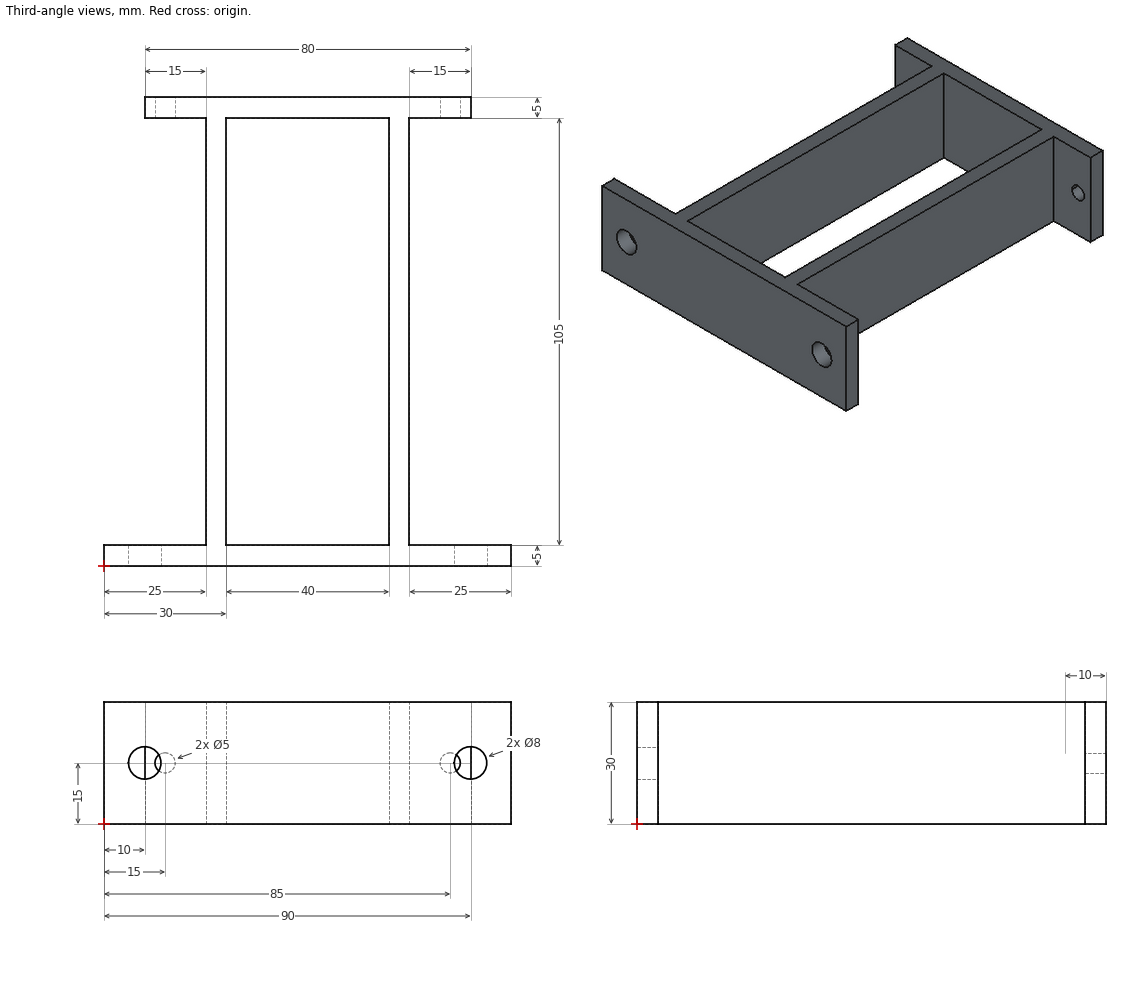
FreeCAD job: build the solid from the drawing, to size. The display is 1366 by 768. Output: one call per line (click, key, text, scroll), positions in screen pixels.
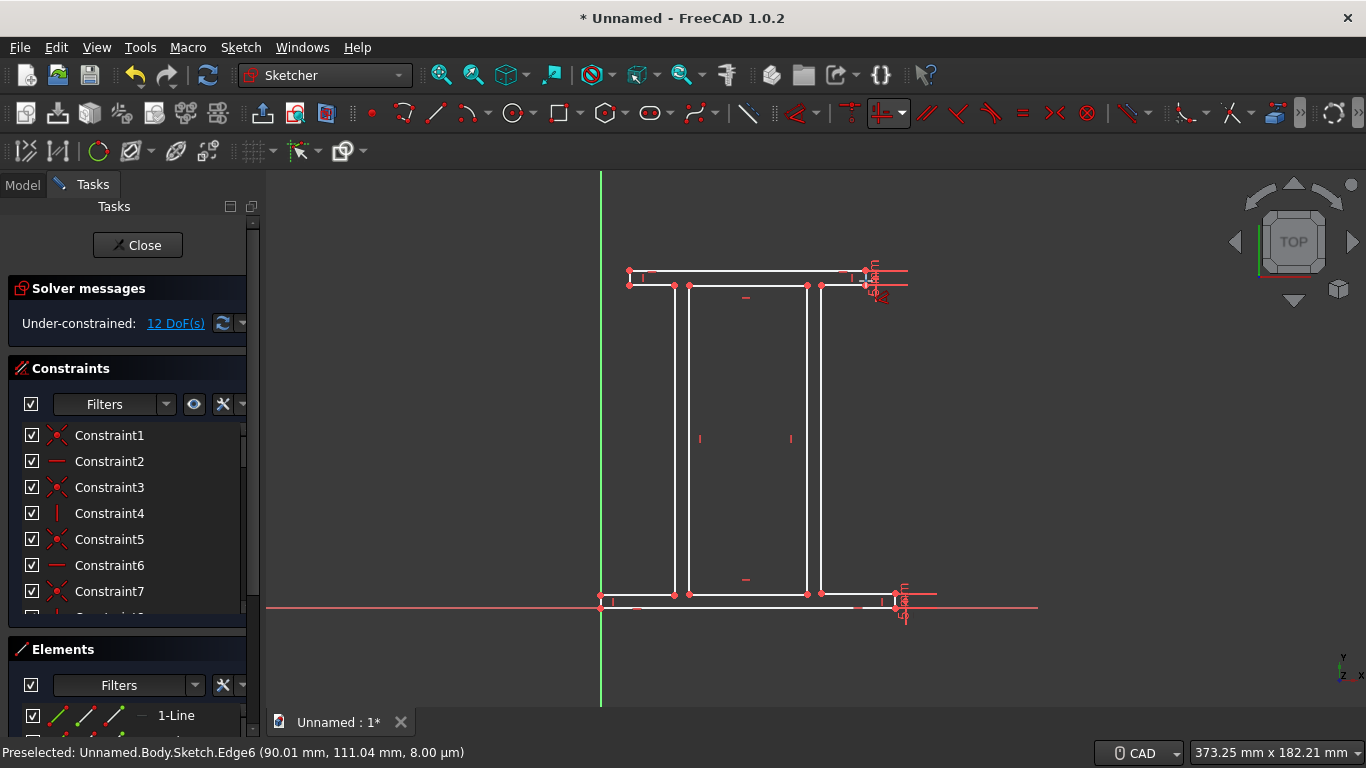
scroll(630, 275, up, 6)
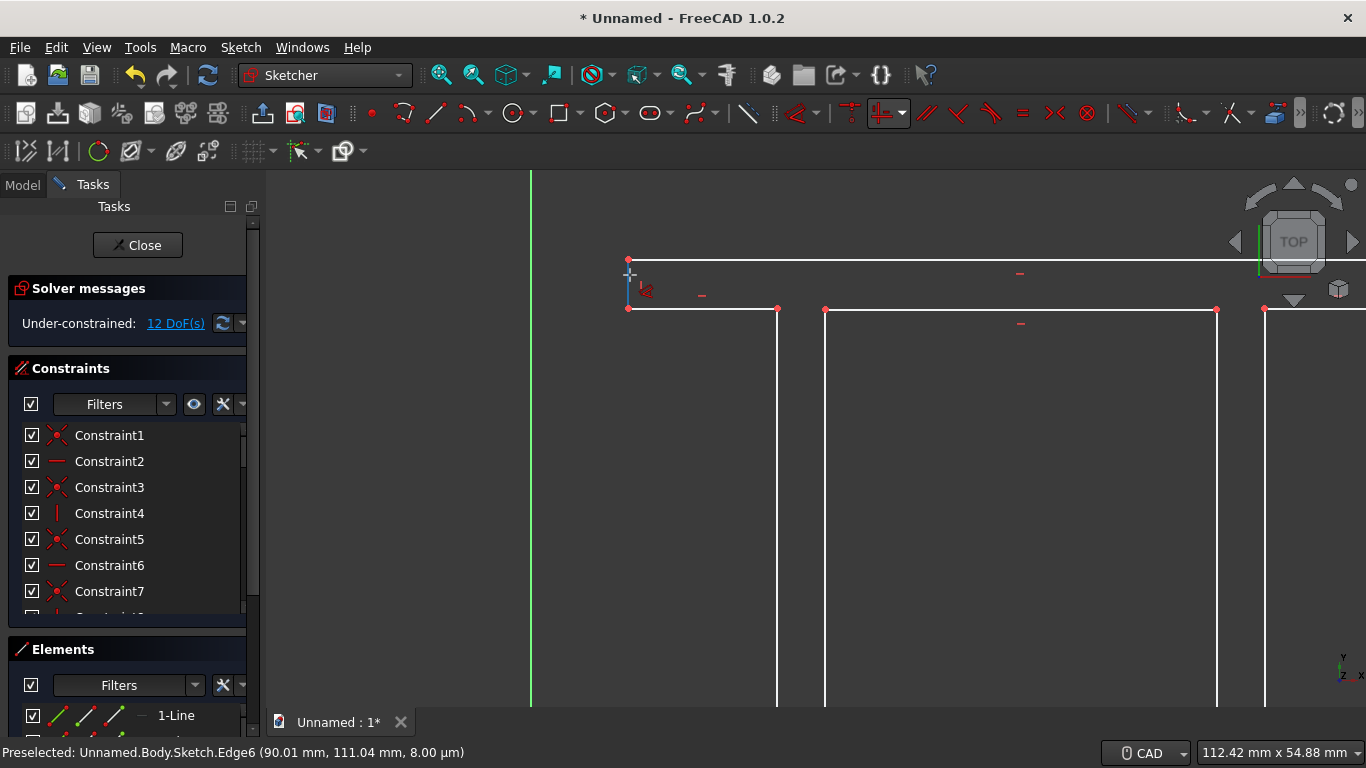
click(628, 274)
click(594, 284)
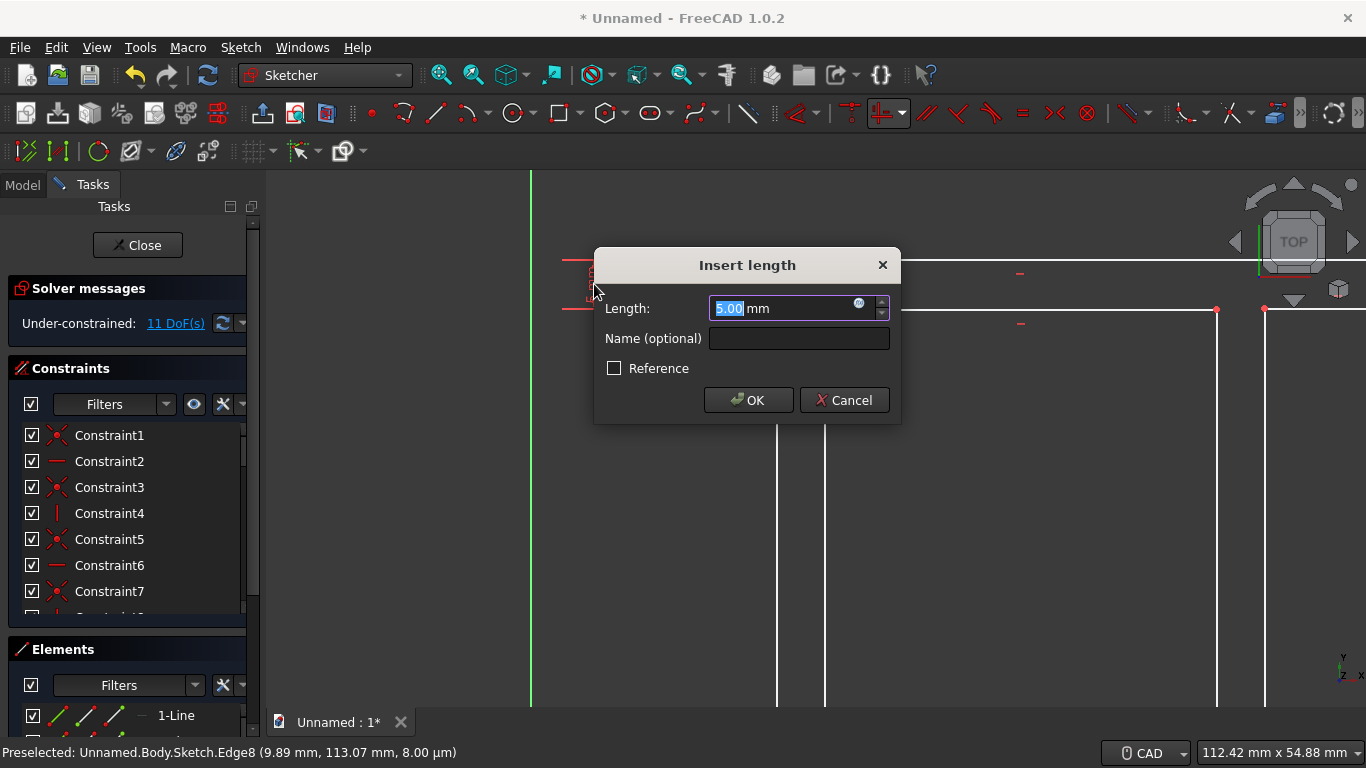
text(5)
key(Return)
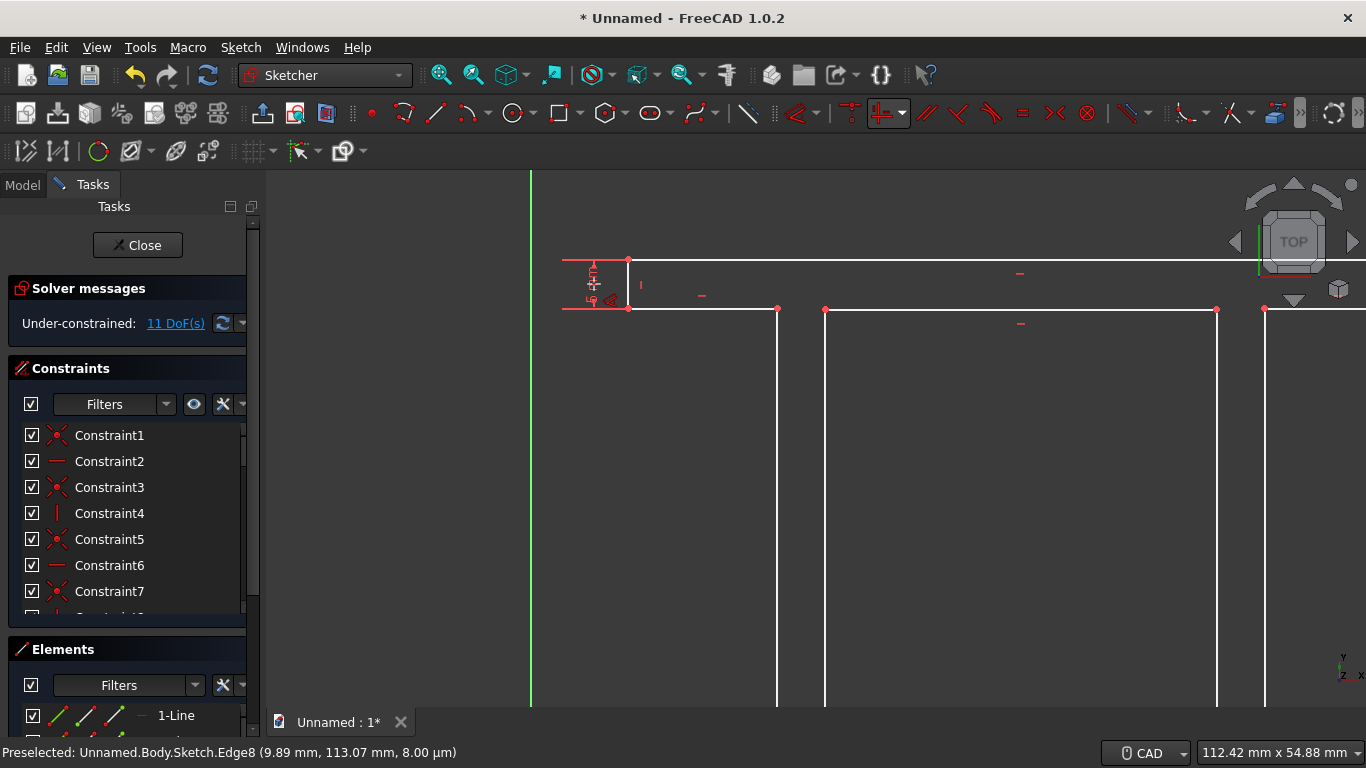
scroll(630, 275, down, 6)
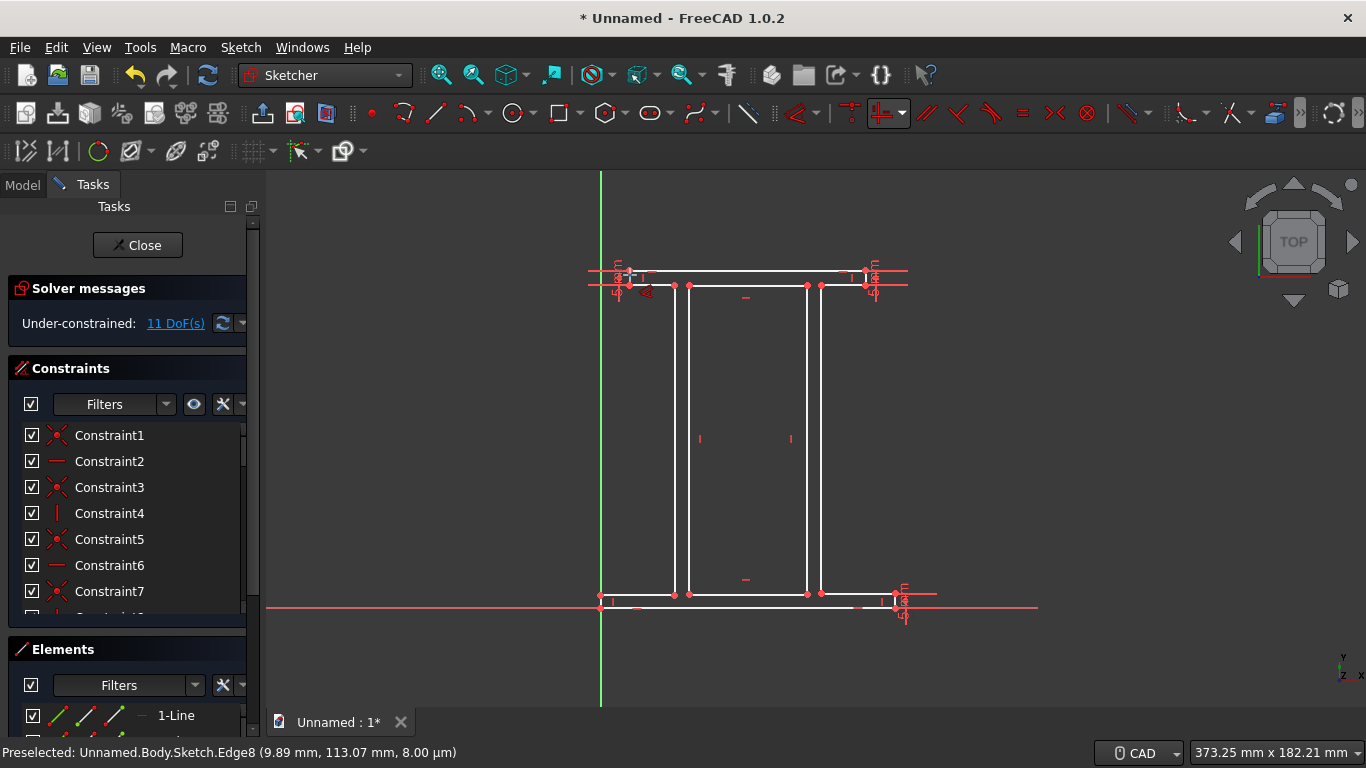
scroll(601, 599, up, 7)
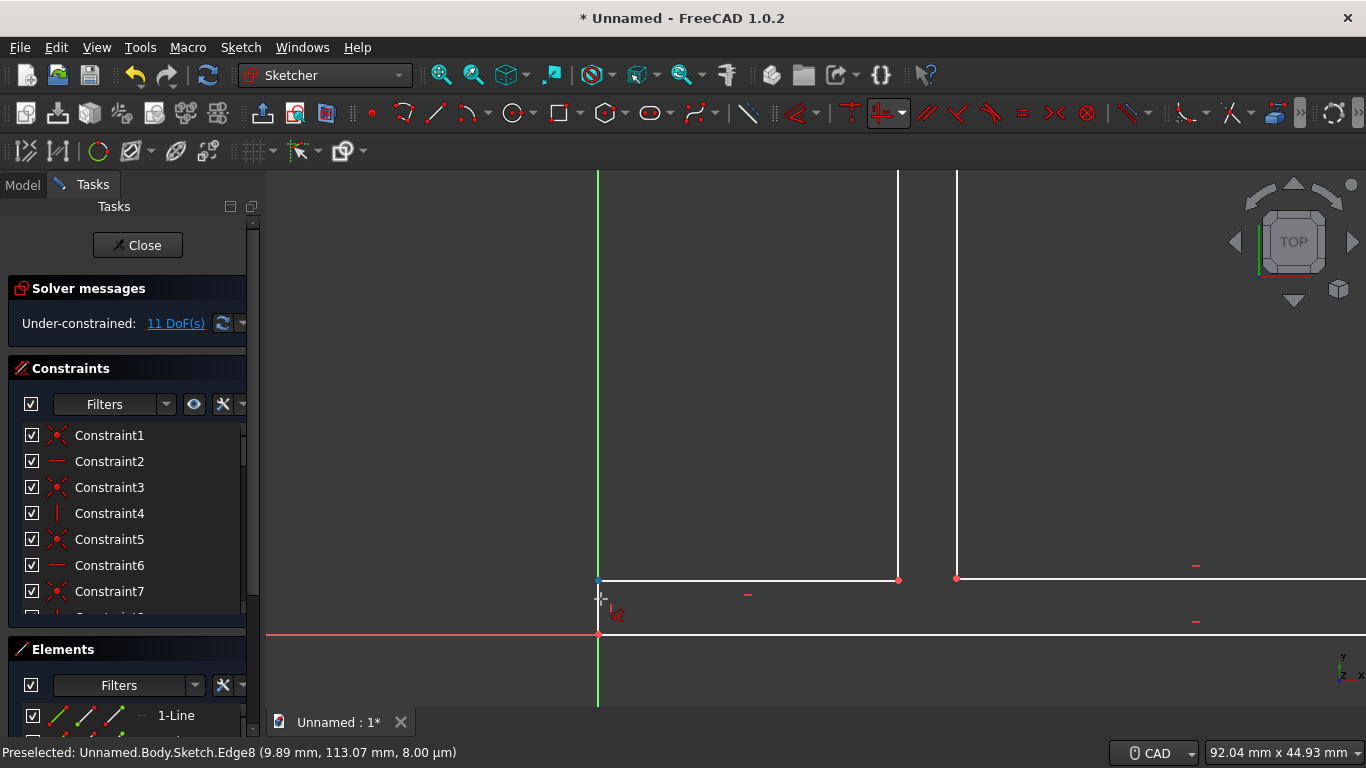
click(598, 597)
click(564, 608)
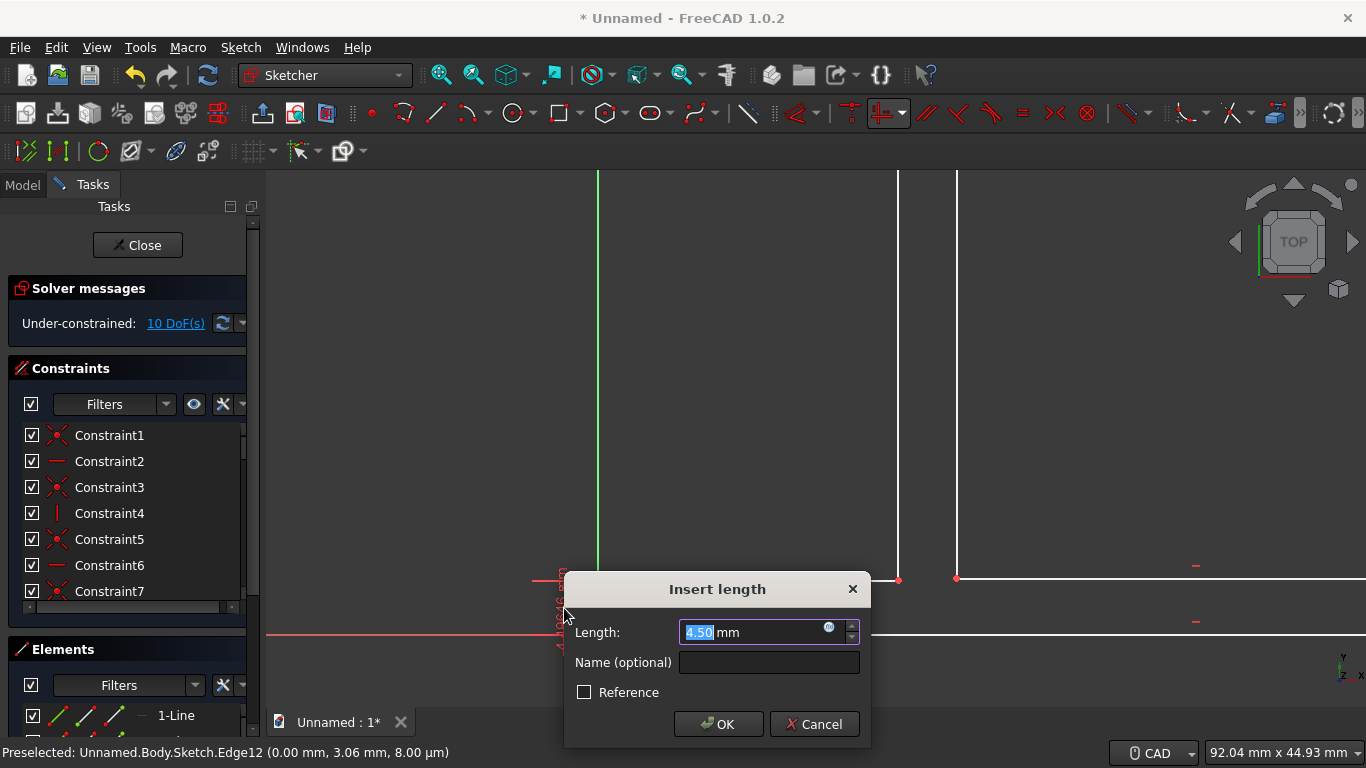
text(5)
key(Return)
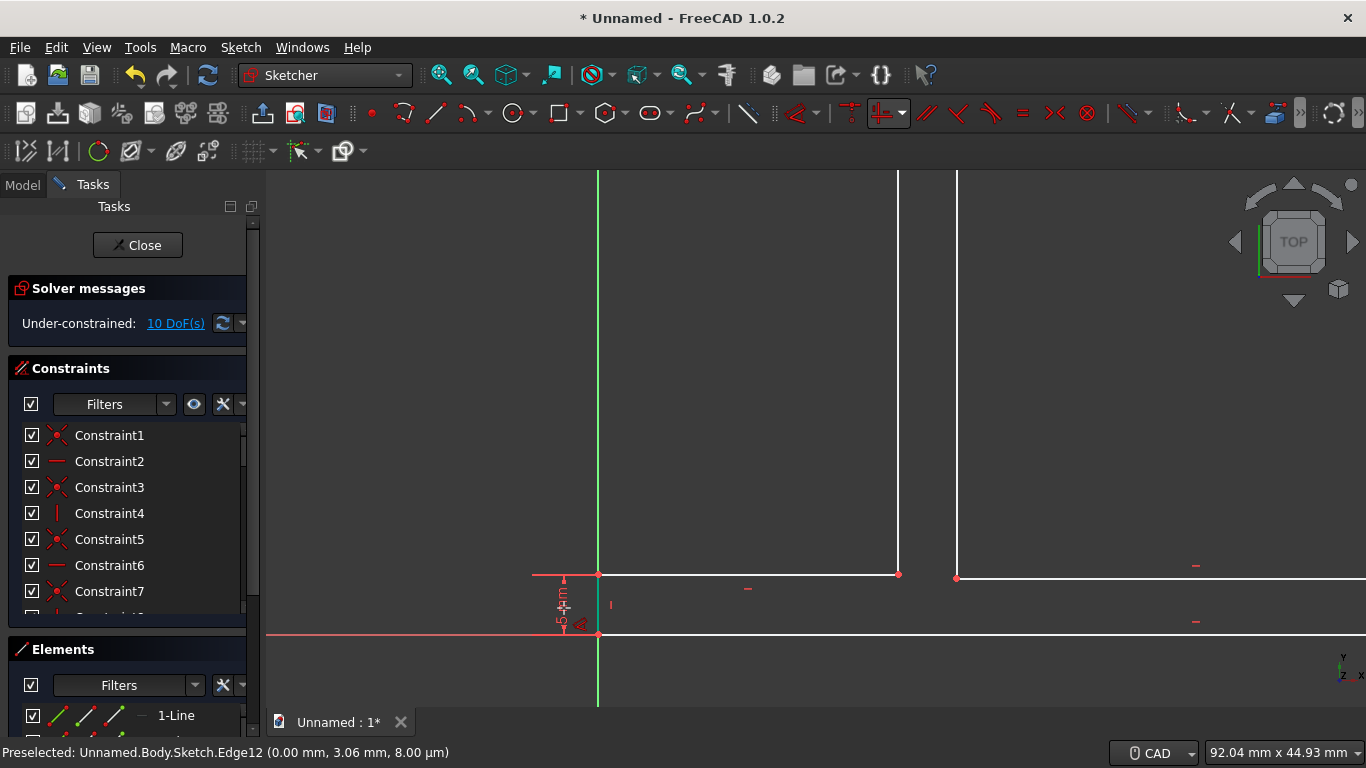
scroll(601, 599, down, 7)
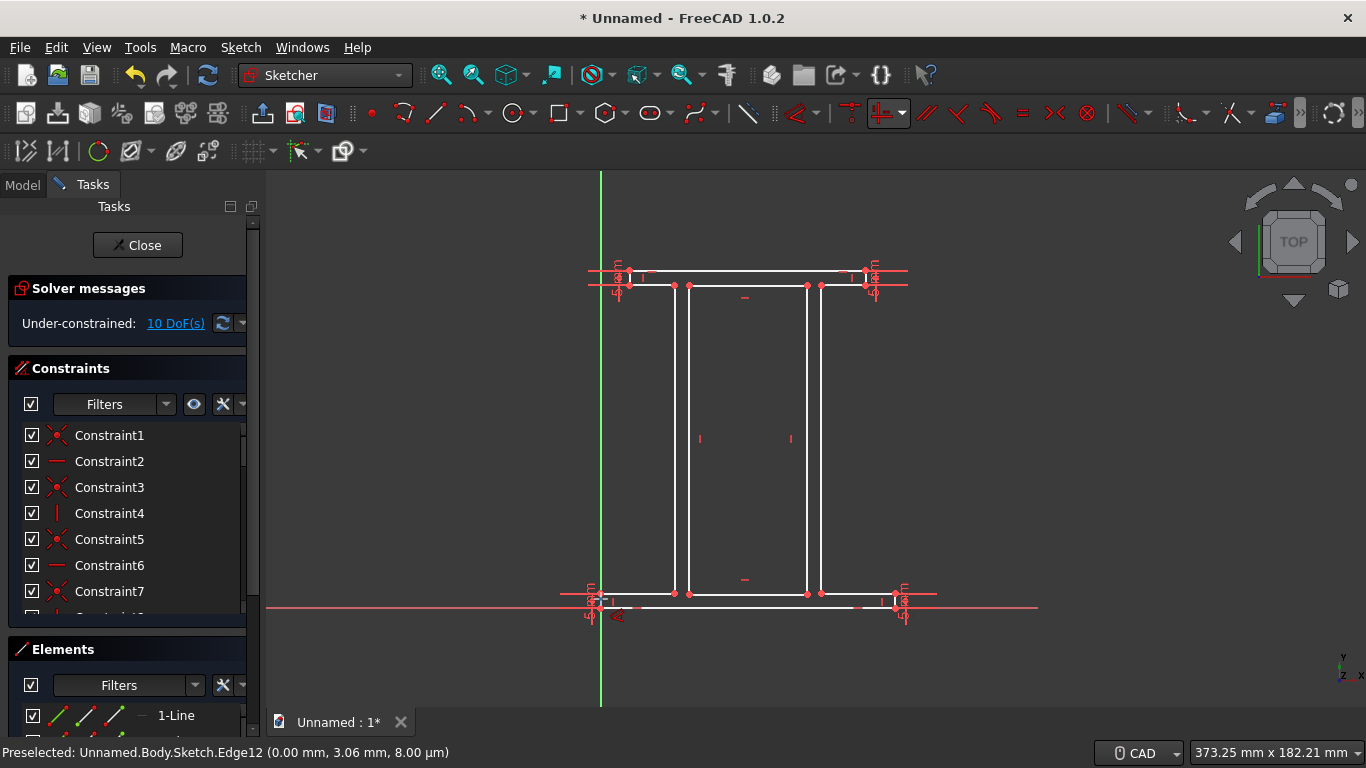
click(873, 594)
click(858, 628)